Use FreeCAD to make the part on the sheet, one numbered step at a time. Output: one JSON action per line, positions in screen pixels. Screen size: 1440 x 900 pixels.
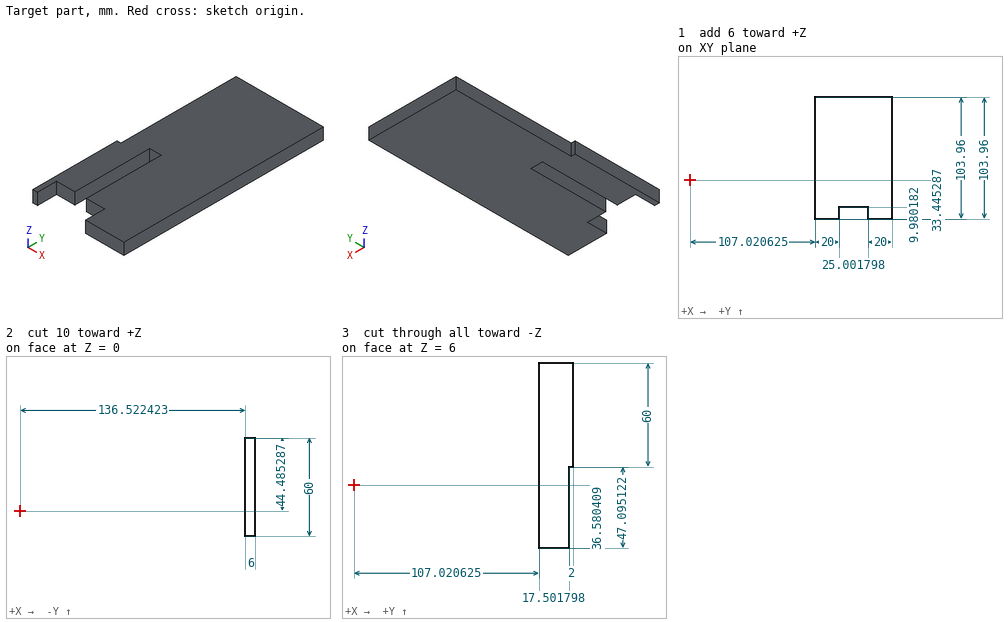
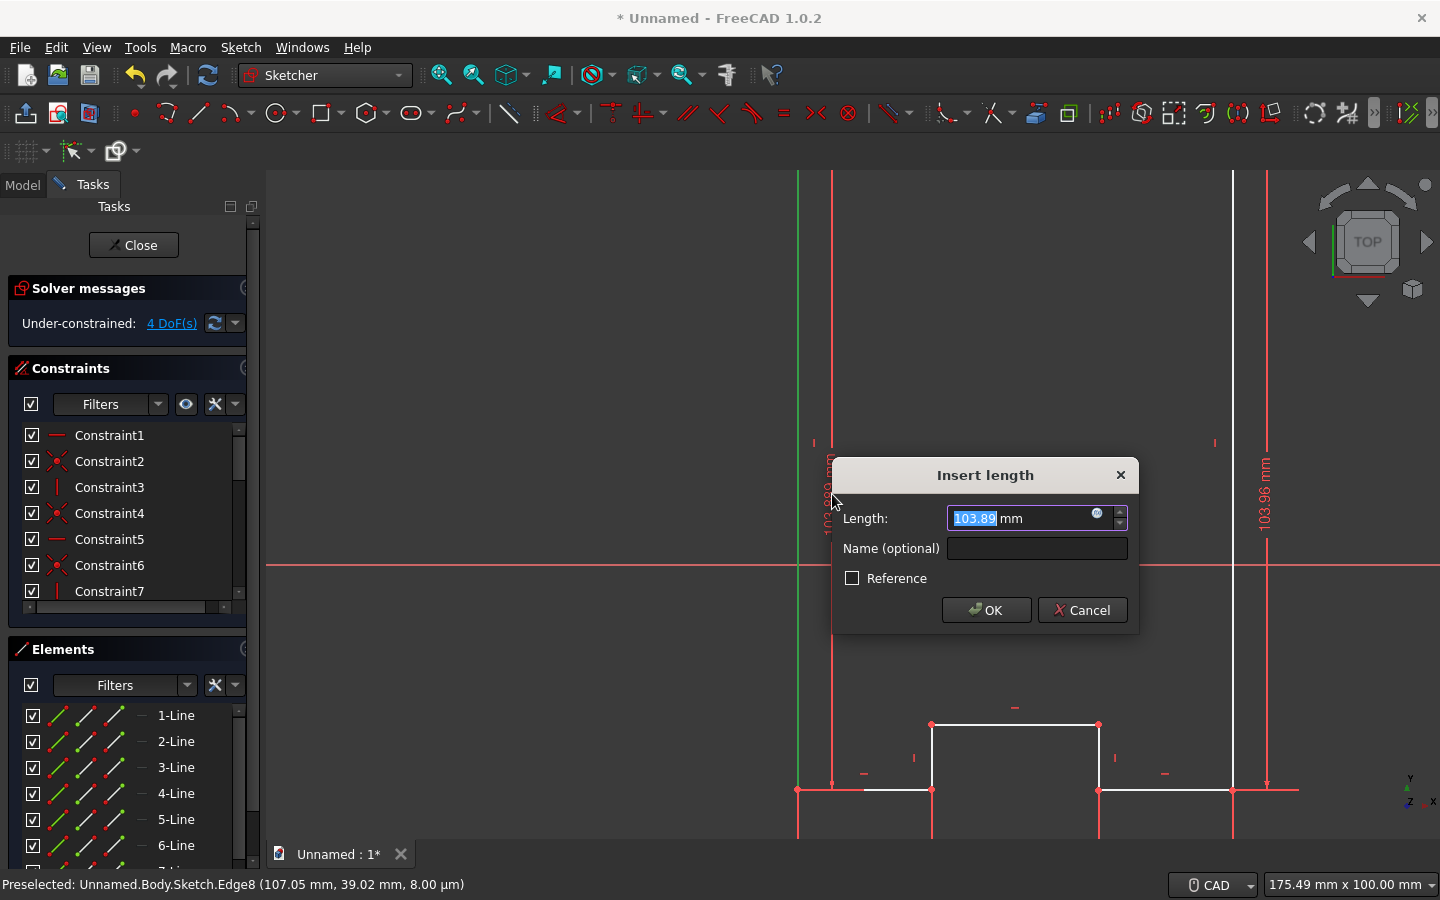
{"action": "type", "text": "103.96"}
{"action": "key", "text": "Return"}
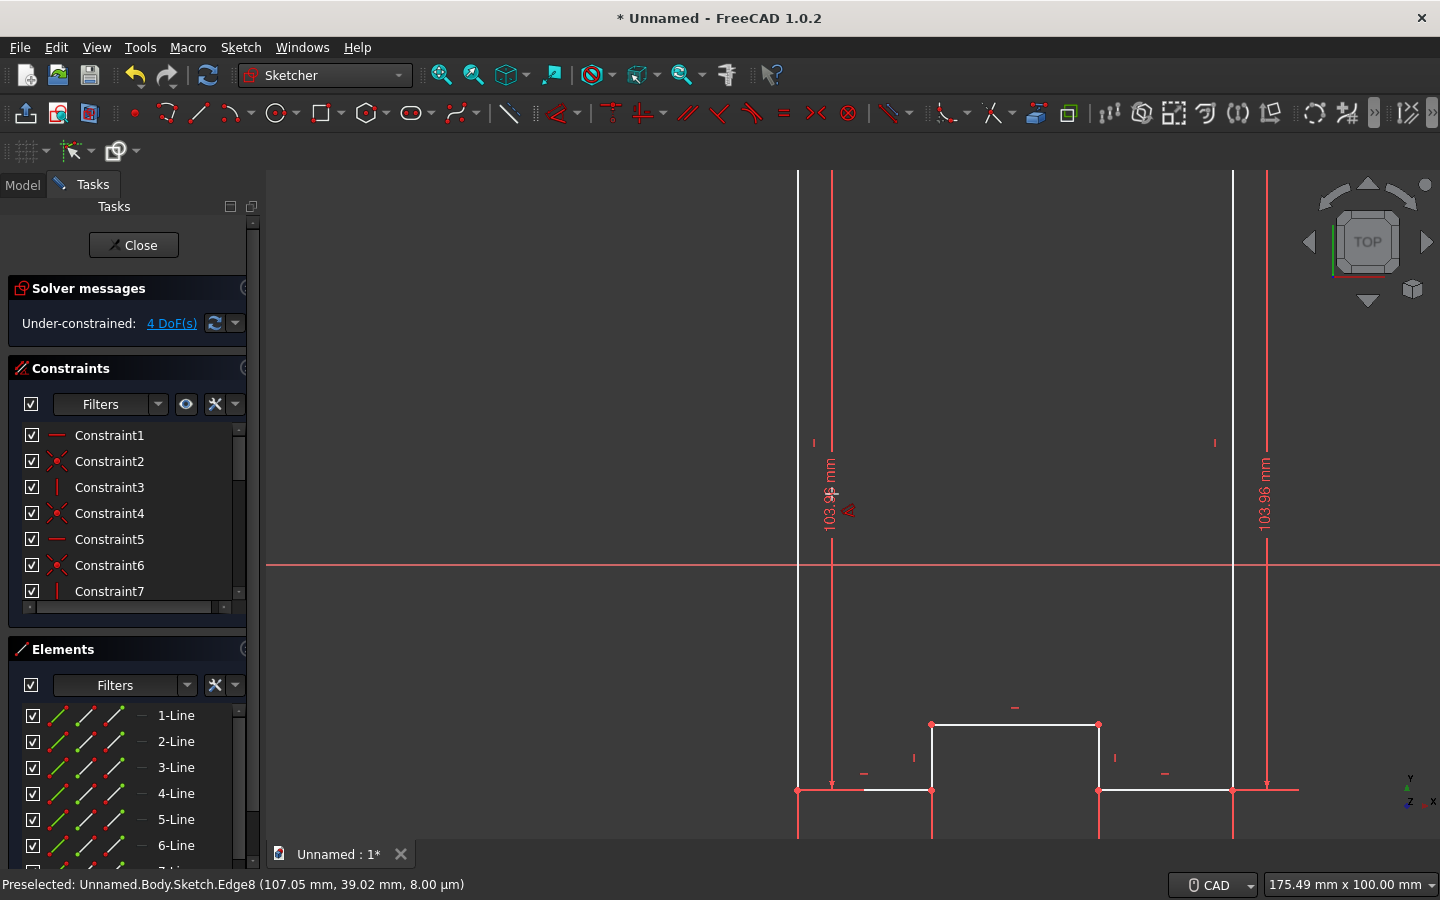
{"action": "left_click", "coordinate": [932, 771]}
{"action": "left_click", "coordinate": [966, 758]}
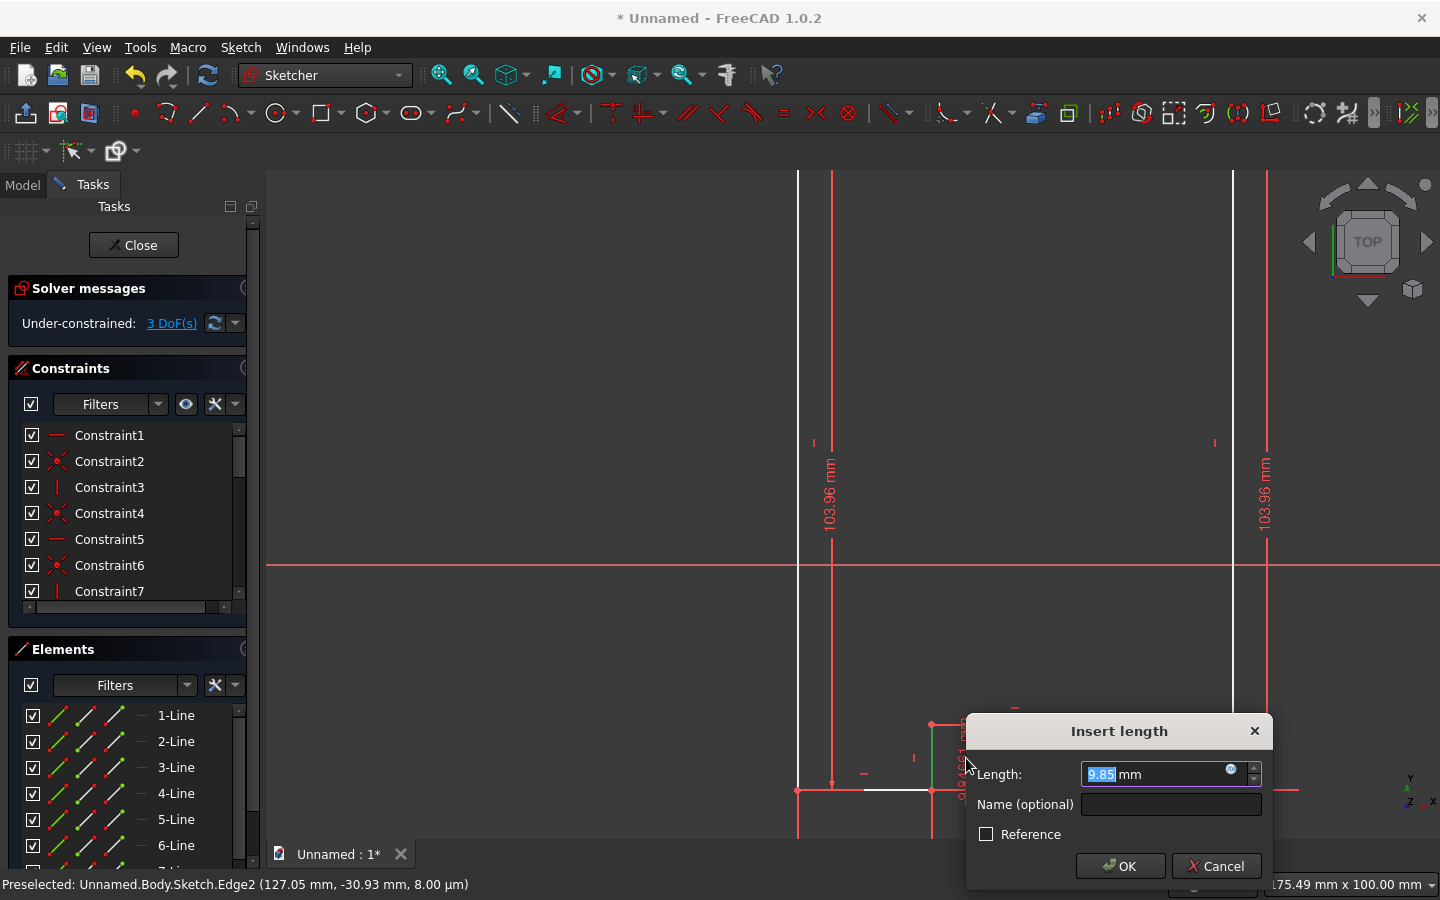
{"action": "type", "text": "9.980182"}
{"action": "key", "text": "Return"}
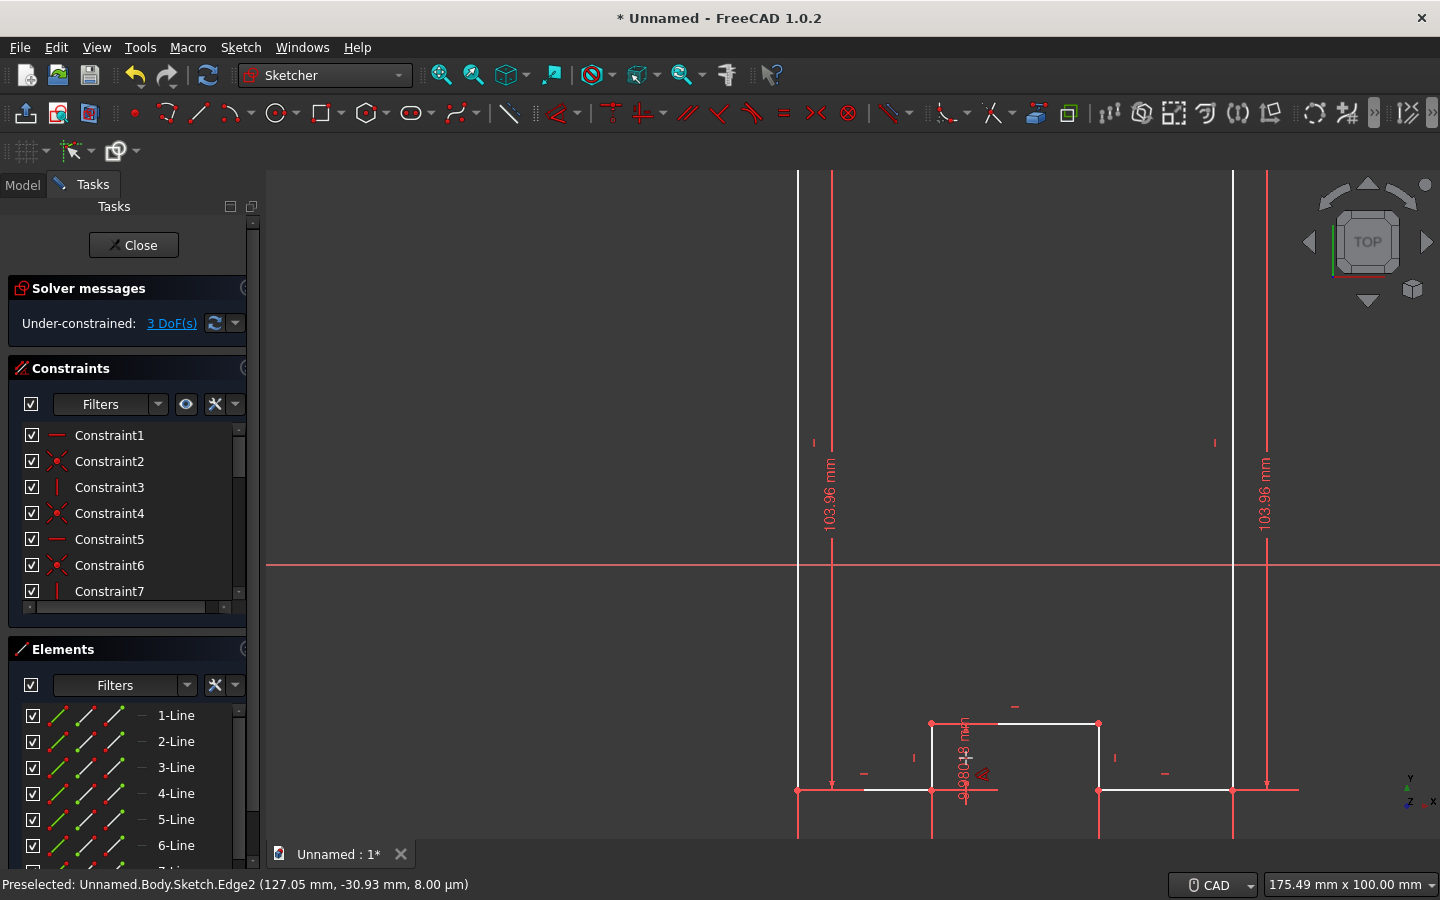
{"action": "left_click", "coordinate": [982, 724]}
{"action": "left_click", "coordinate": [1054, 758]}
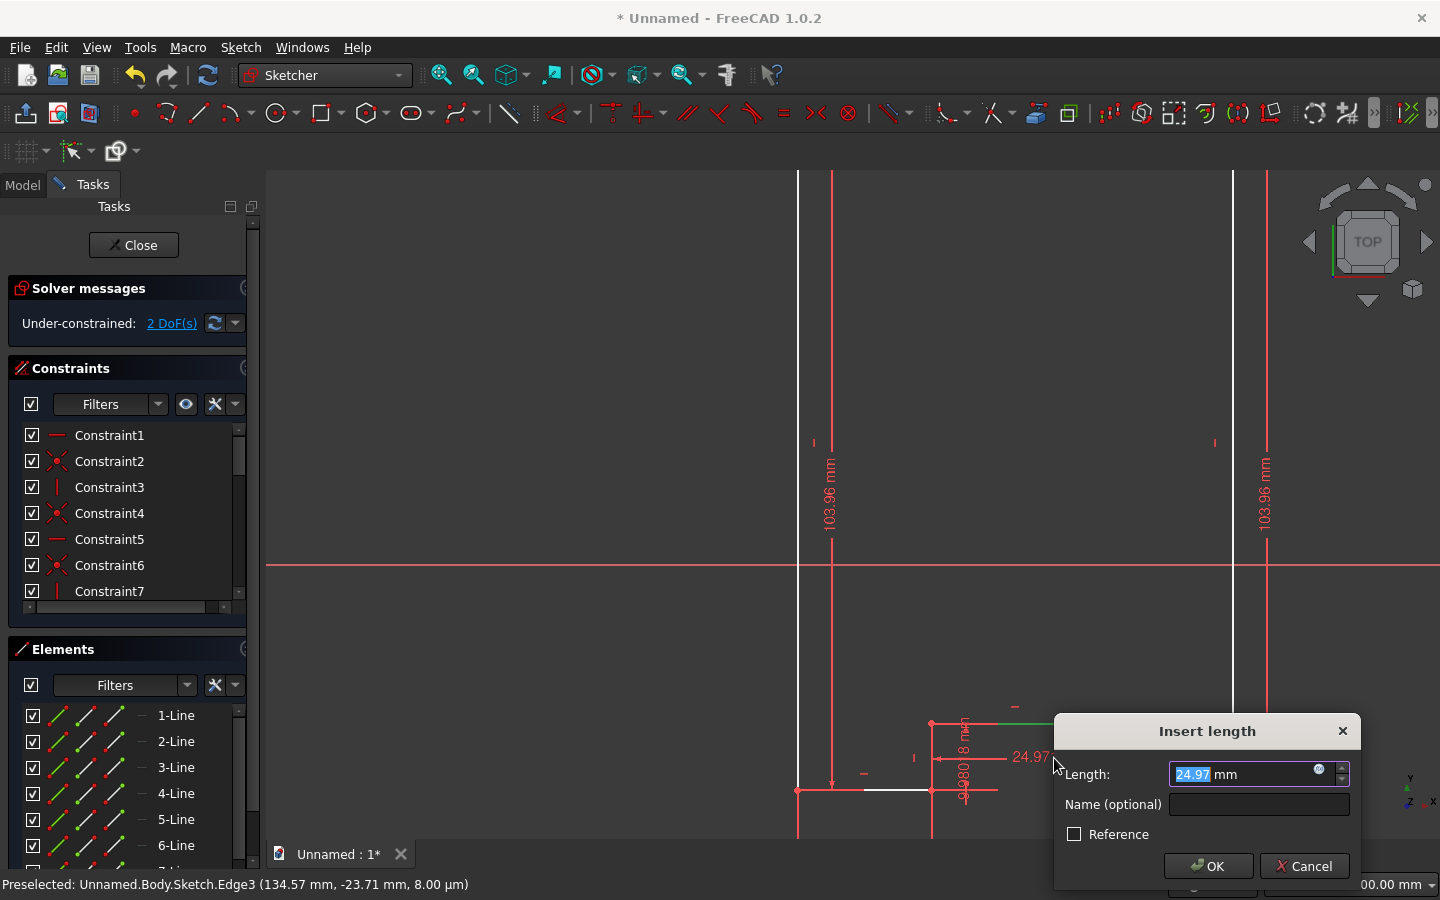
{"action": "type", "text": "25.001798"}
{"action": "key", "text": "Return"}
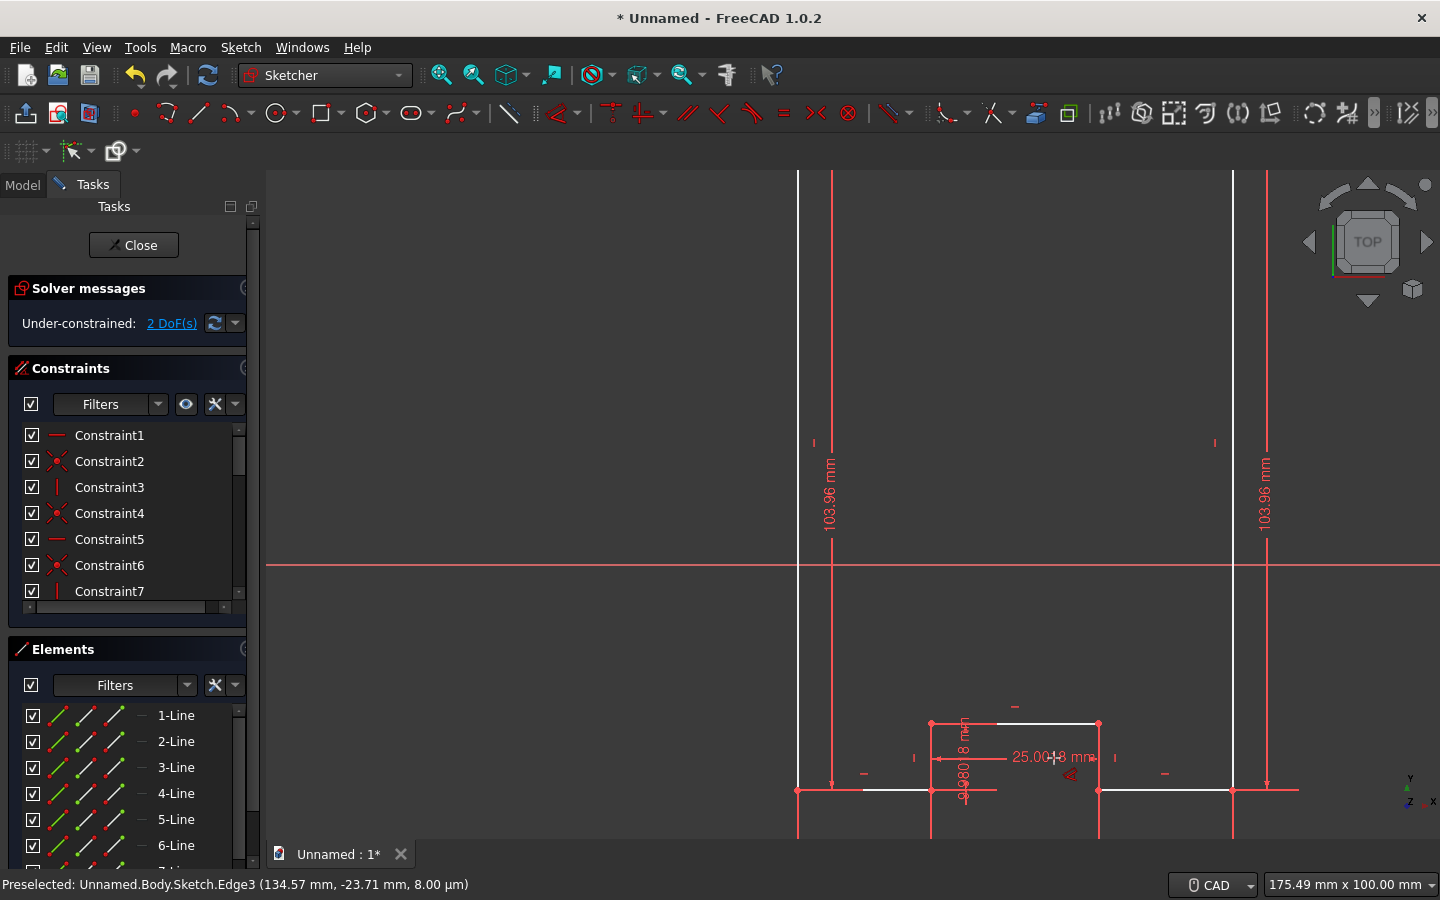
{"action": "left_click", "coordinate": [798, 790]}
{"action": "left_click", "coordinate": [832, 678]}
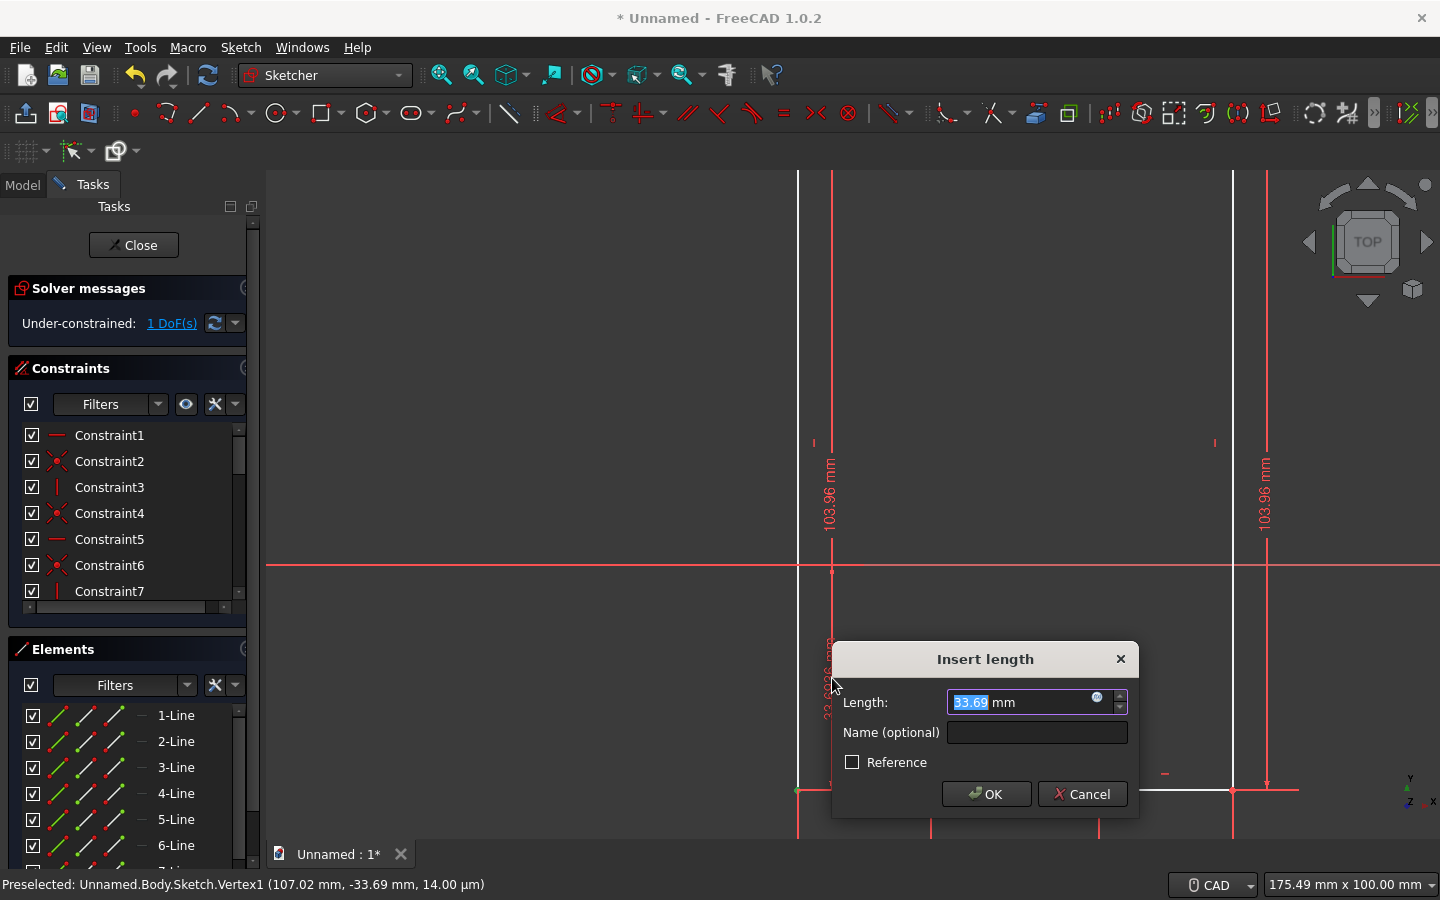
{"action": "type", "text": "33.445287"}
{"action": "key", "text": "Return"}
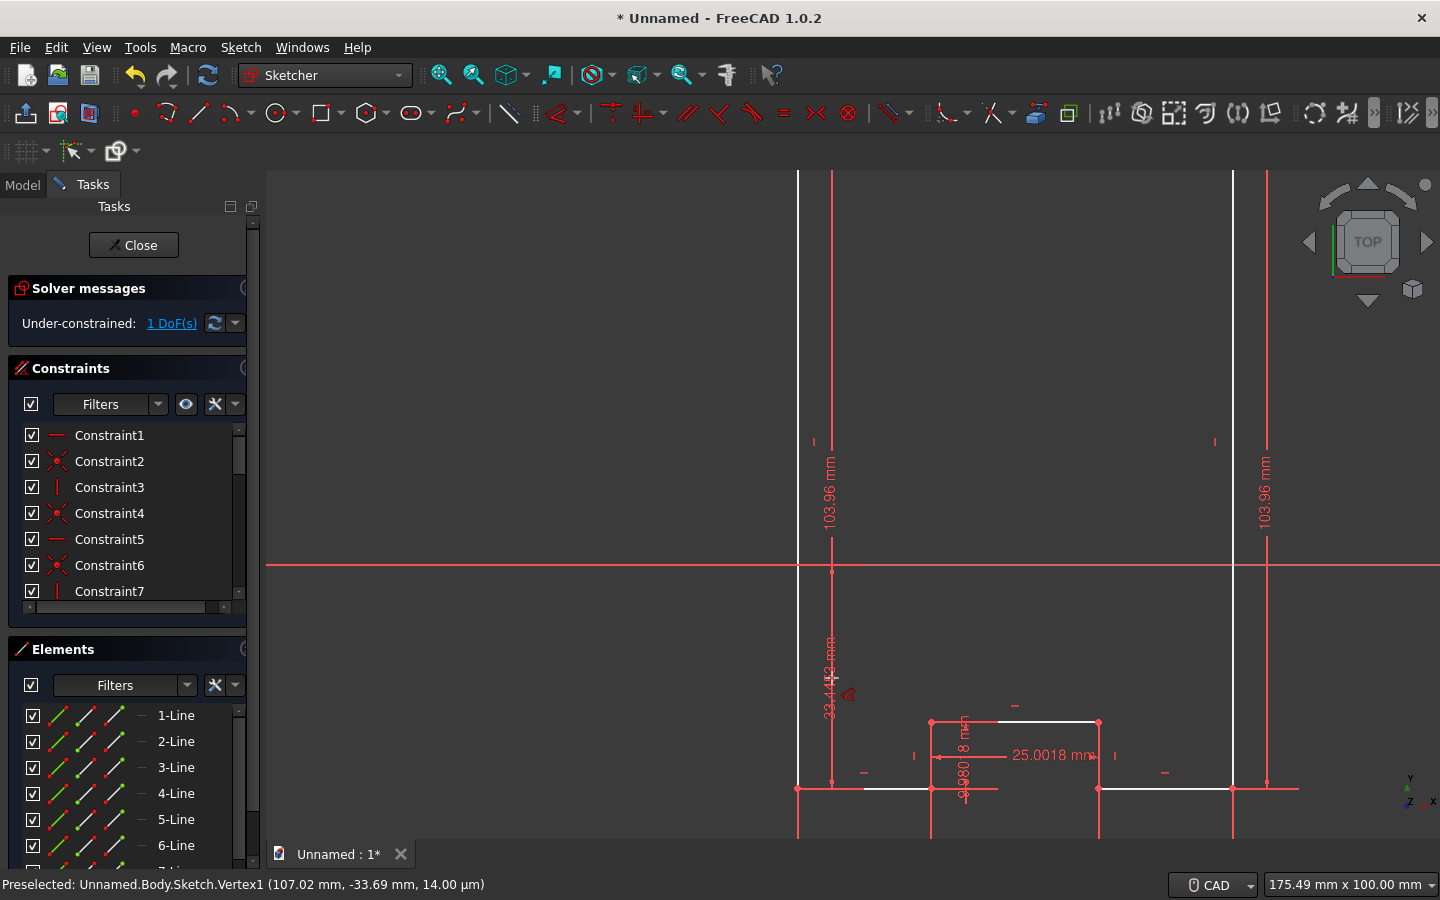
{"action": "left_click", "coordinate": [798, 789]}
{"action": "left_click", "coordinate": [546, 531]}